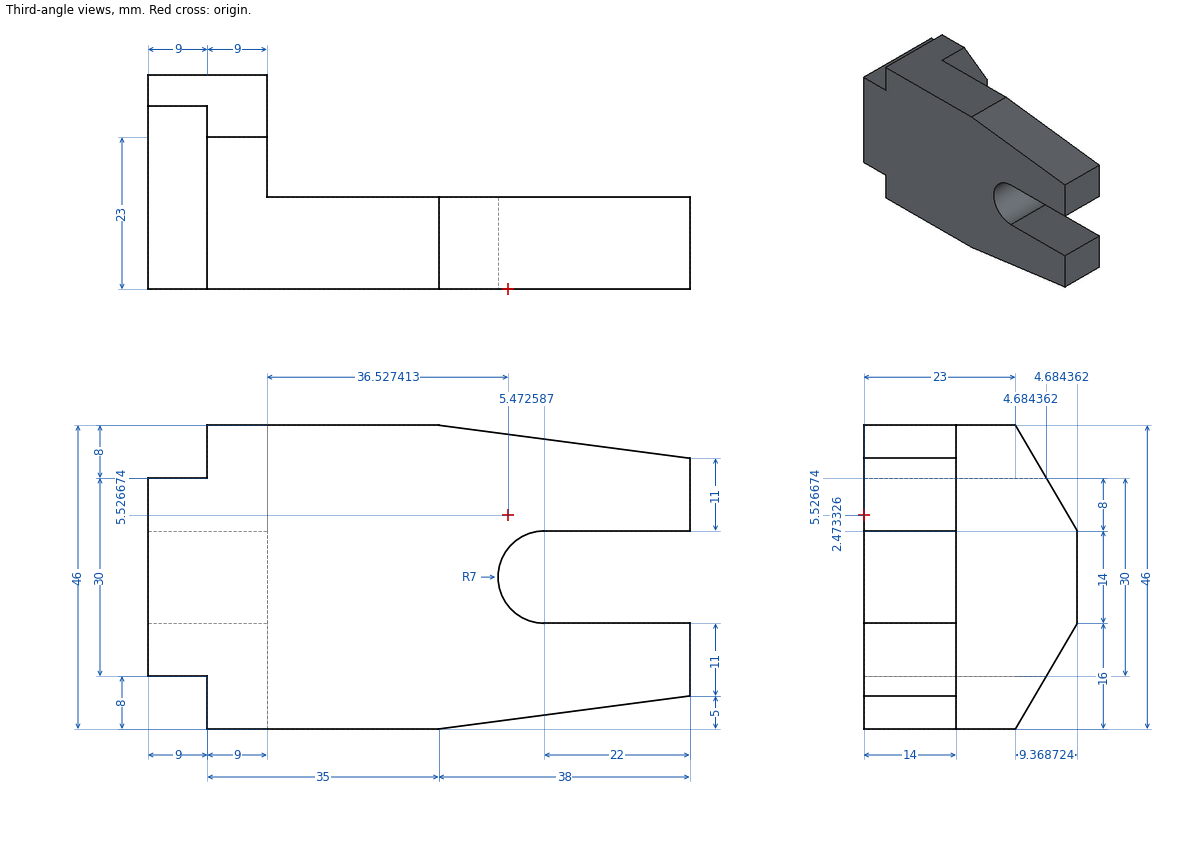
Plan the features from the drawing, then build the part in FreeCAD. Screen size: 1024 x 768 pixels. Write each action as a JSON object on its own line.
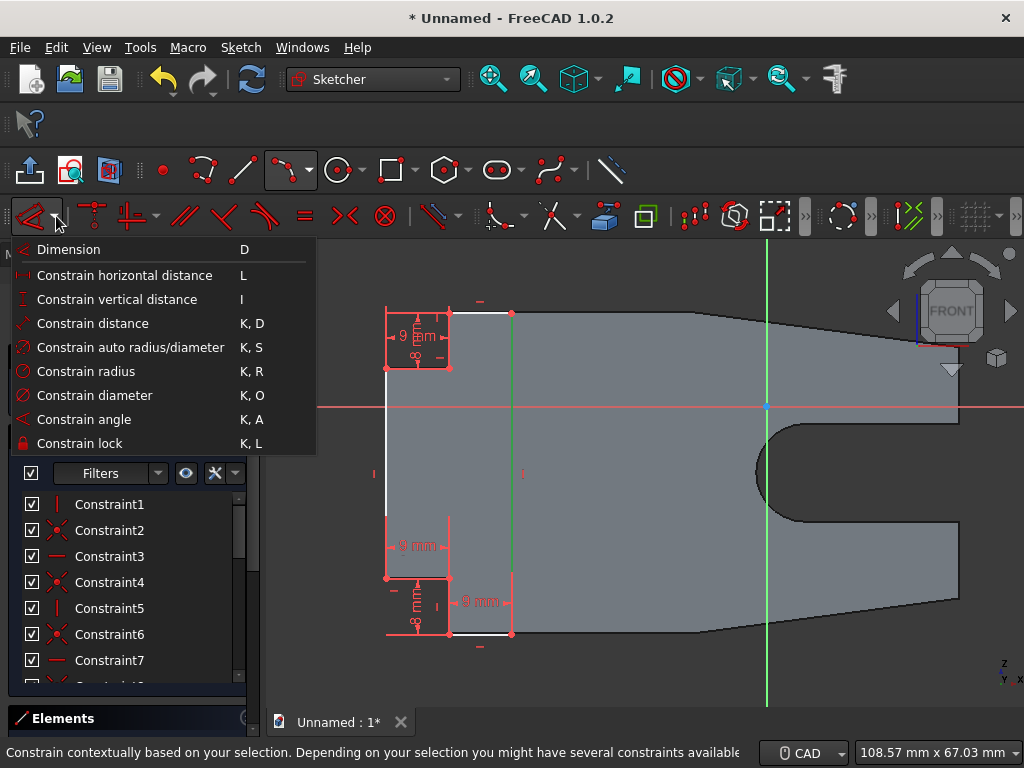
{"action": "left_click", "coordinate": [164, 299]}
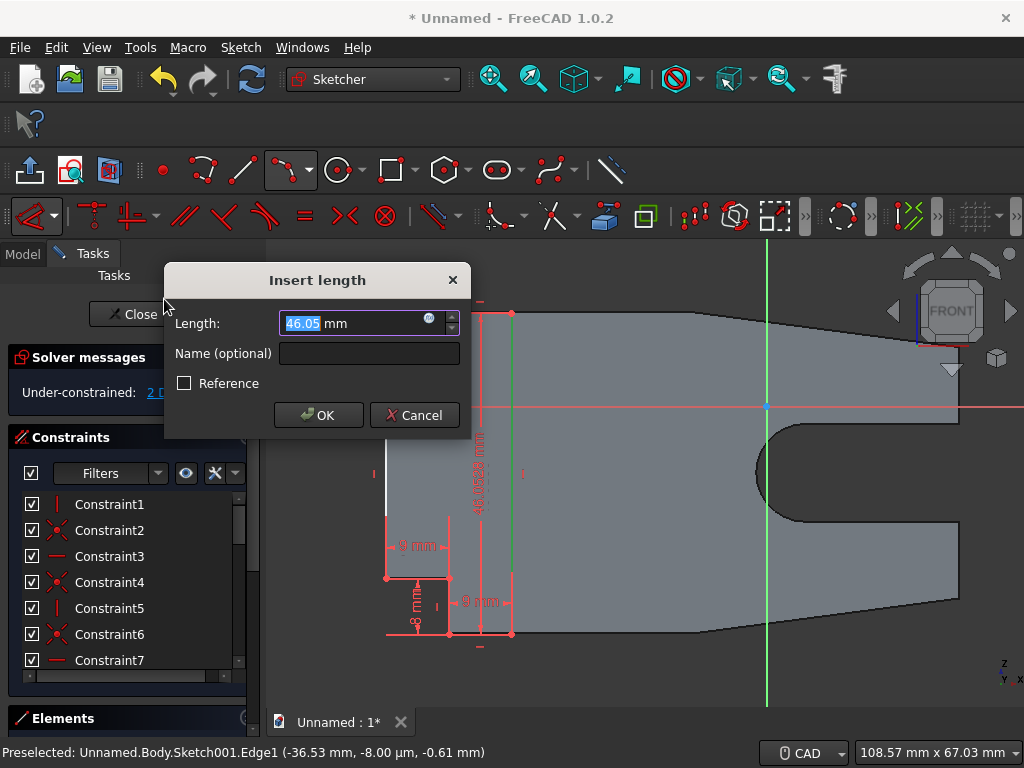
{"action": "type", "text": "46"}
{"action": "key", "text": "Return"}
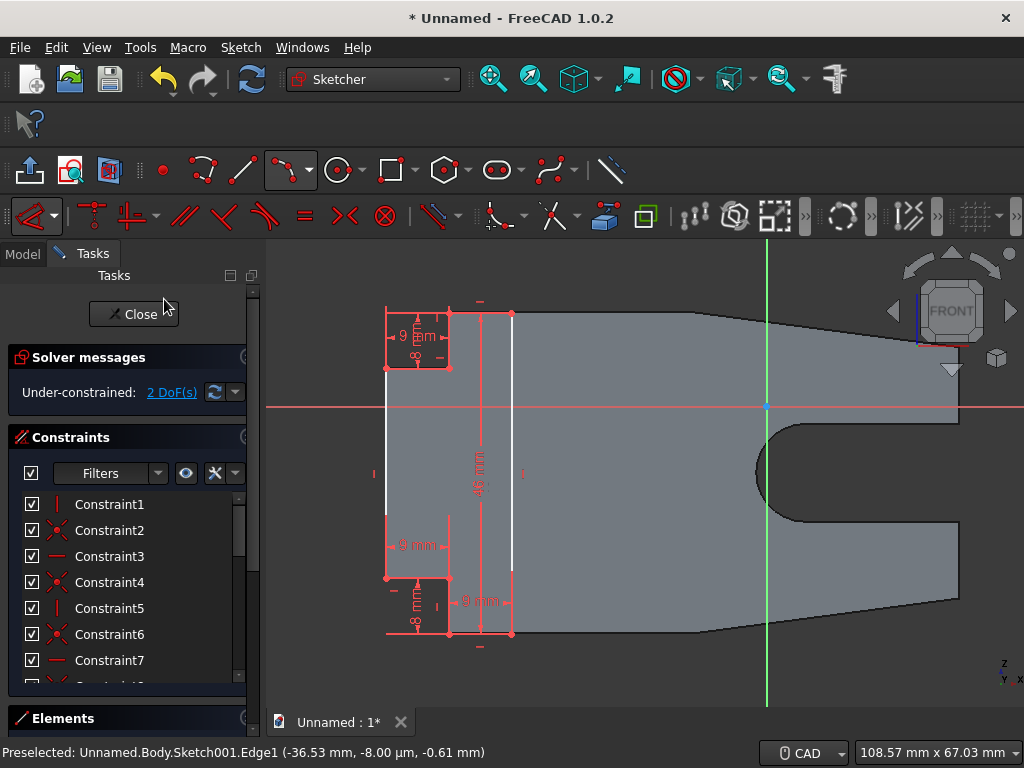
{"action": "left_click", "coordinate": [386, 369]}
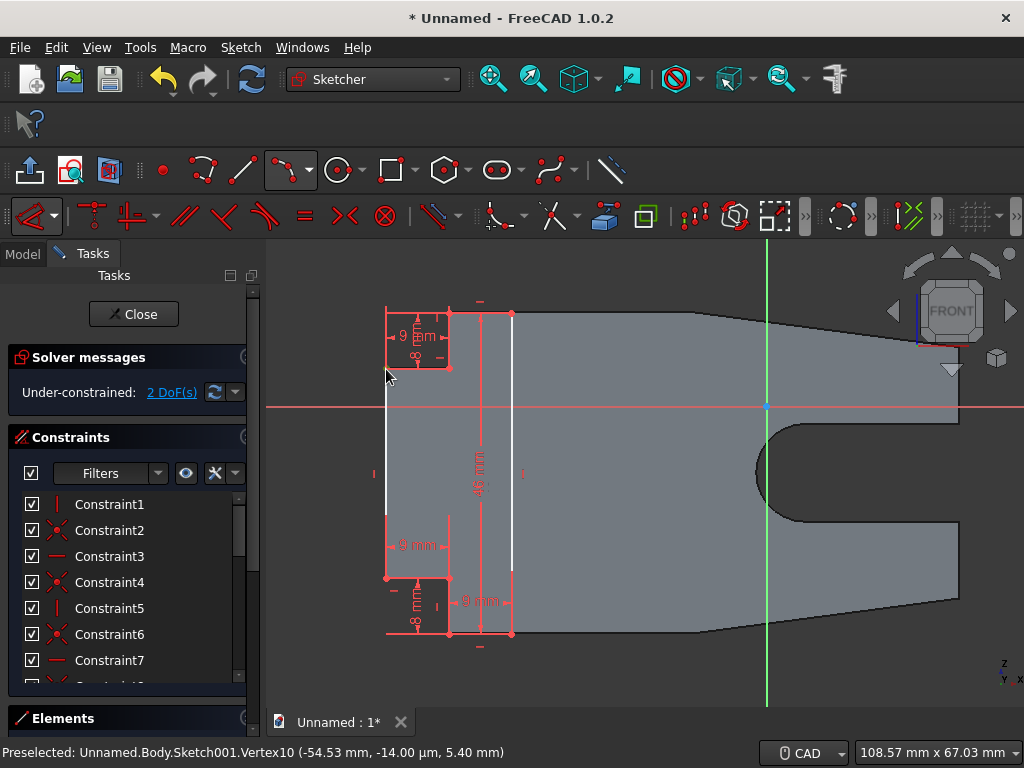
{"action": "key", "text": "i"}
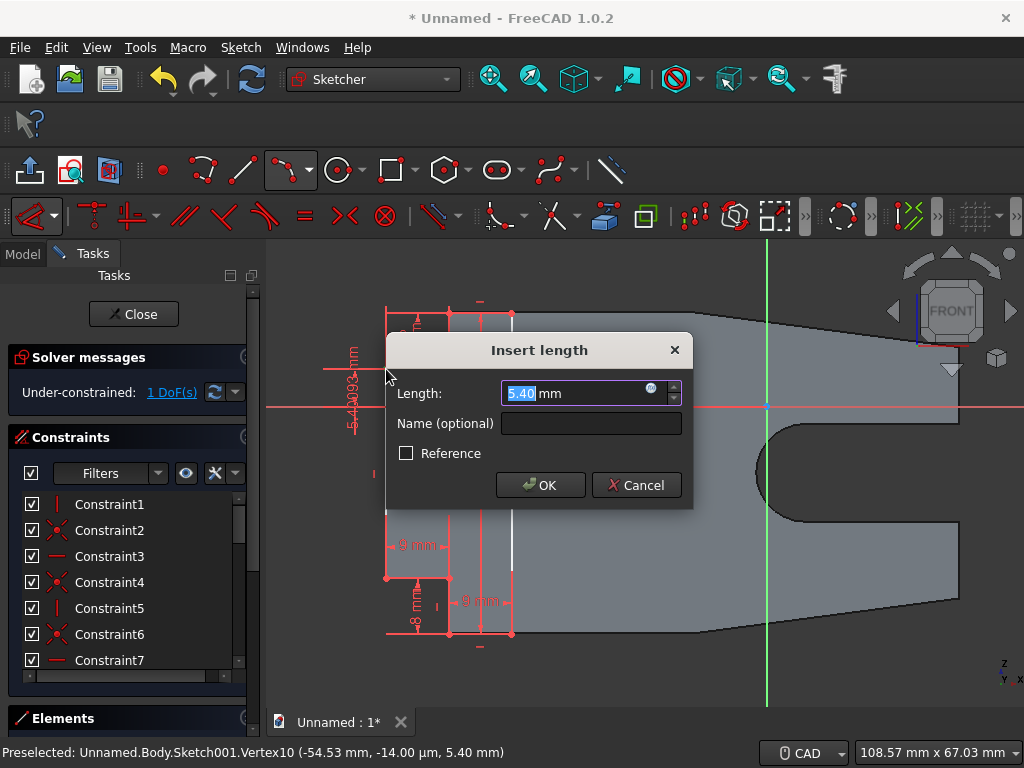
{"action": "type", "text": "5.526674"}
{"action": "key", "text": "Return"}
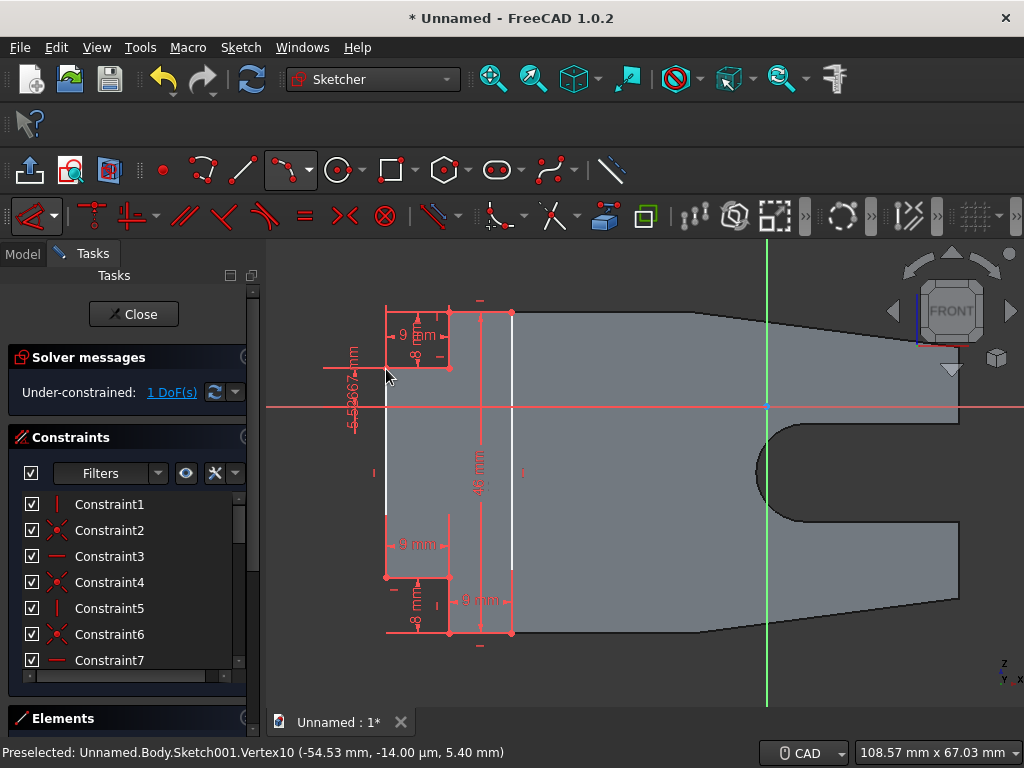
{"action": "left_click", "coordinate": [512, 312]}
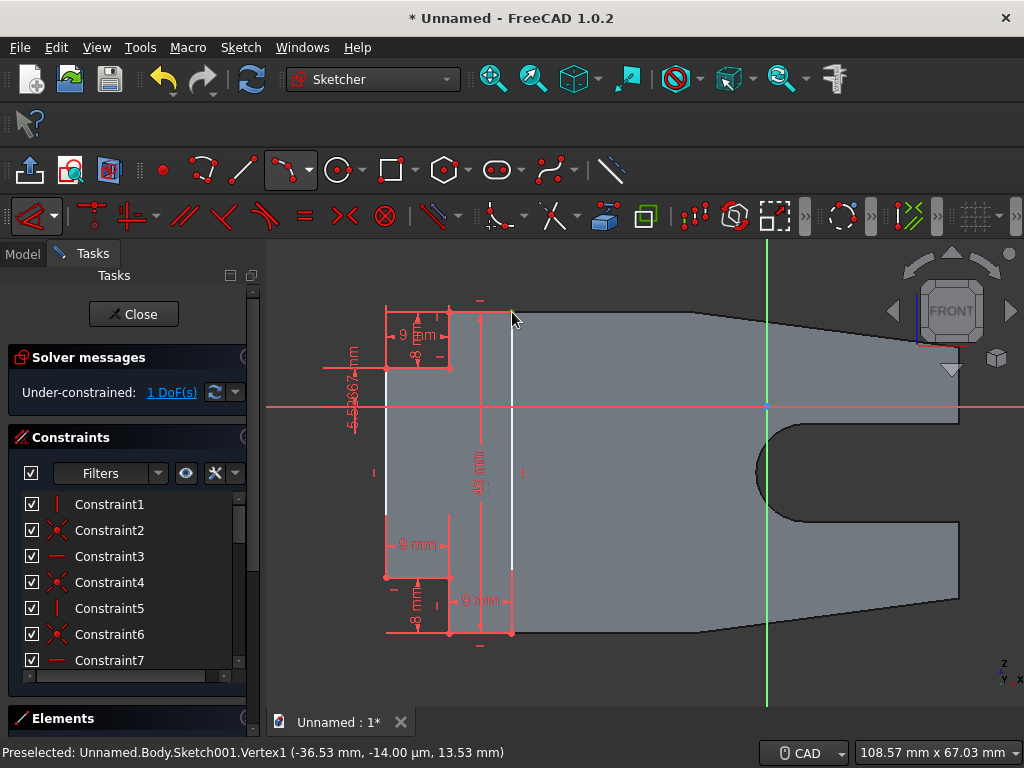
{"action": "left_click", "coordinate": [56, 216]}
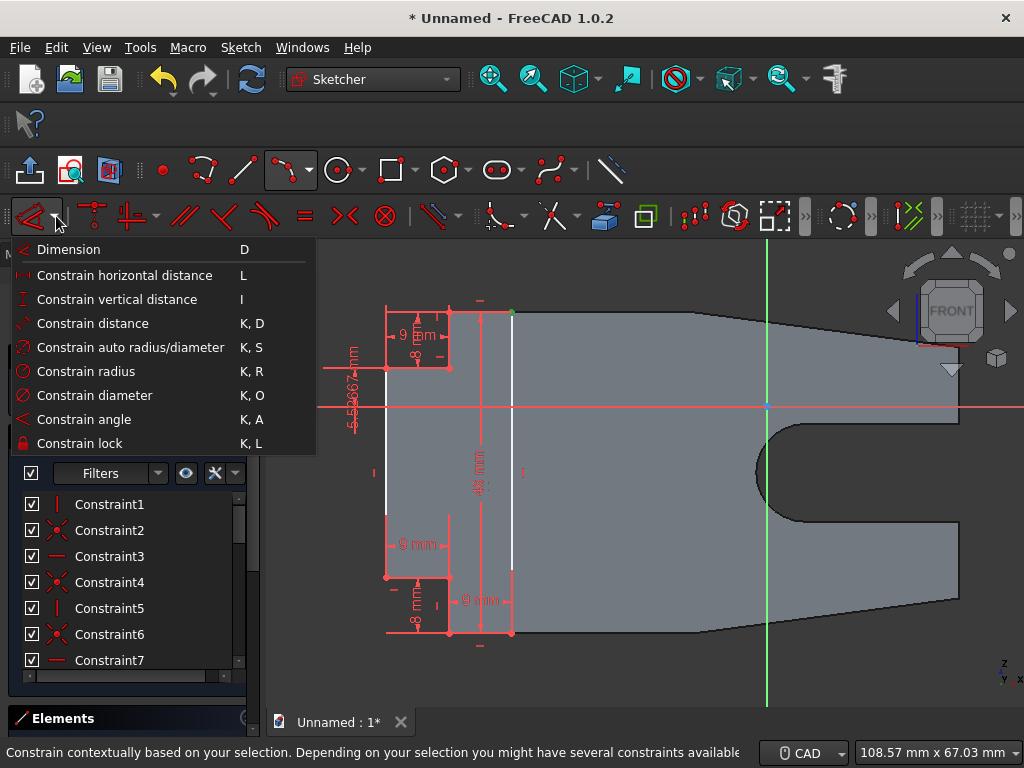
{"action": "left_click", "coordinate": [164, 275]}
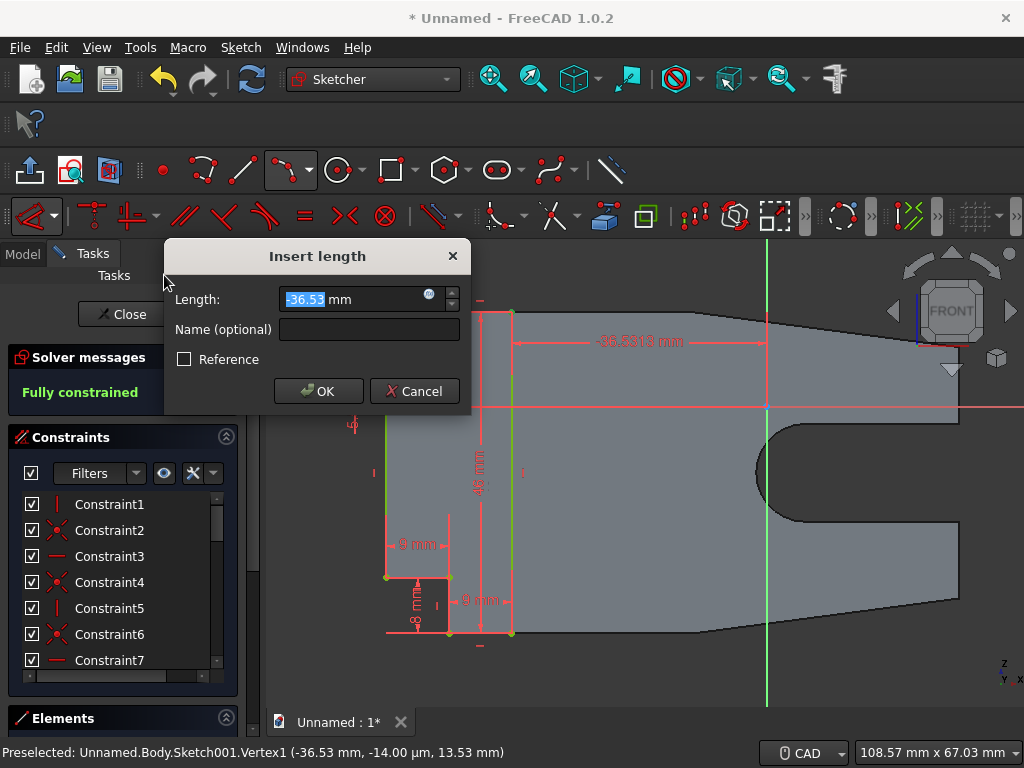
{"action": "type", "text": "-36.527413"}
{"action": "key", "text": "Return"}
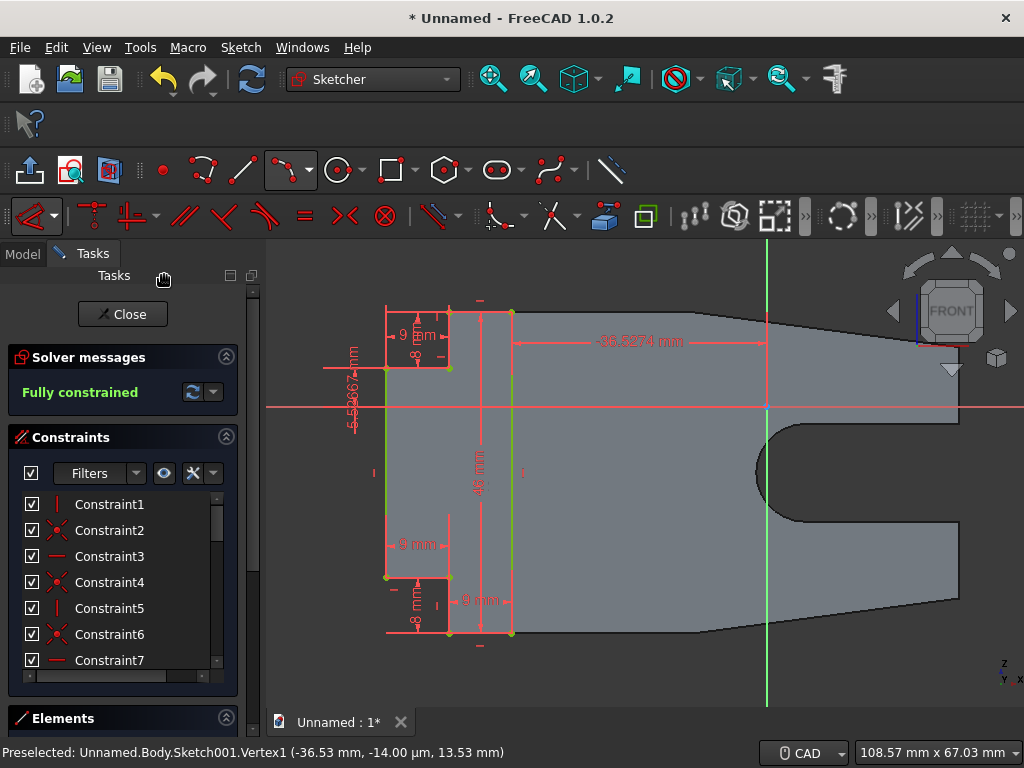
{"action": "left_click", "coordinate": [123, 314]}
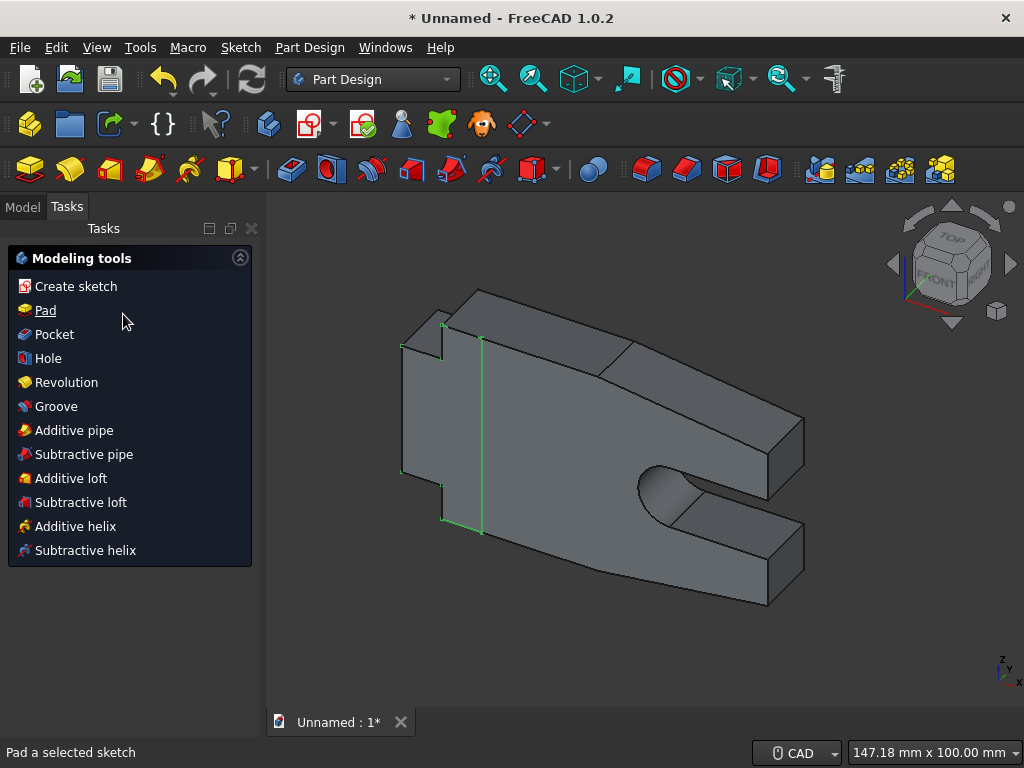
{"action": "left_click", "coordinate": [30, 170]}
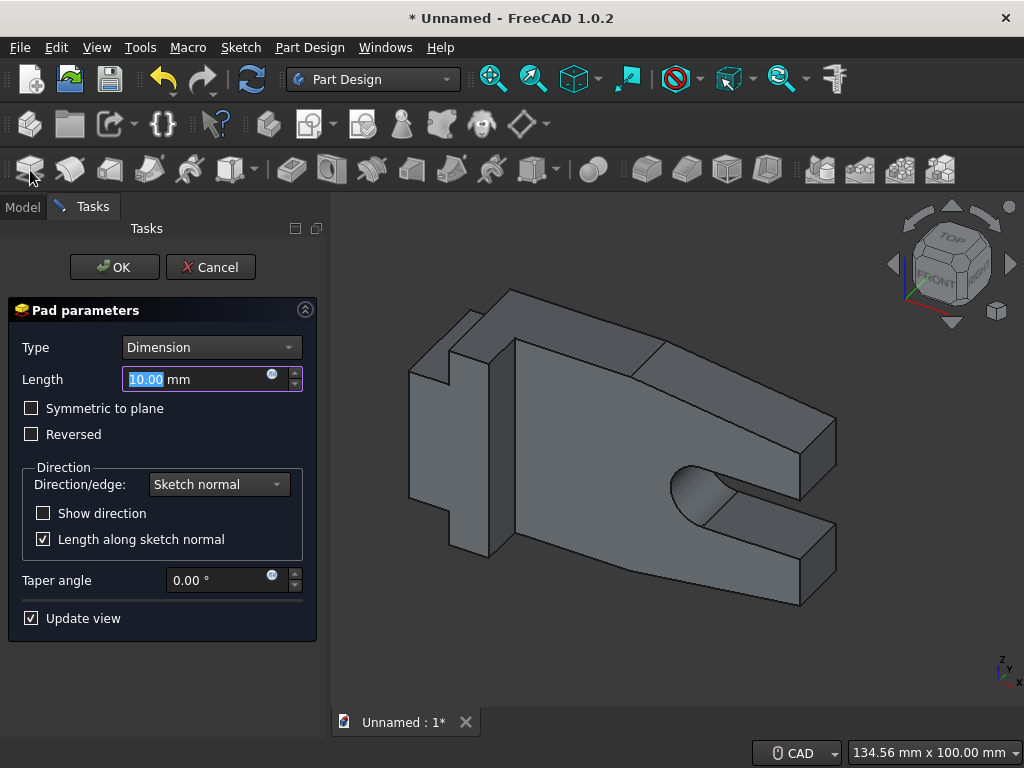
{"action": "type", "text": "23"}
{"action": "key", "text": "Tab"}